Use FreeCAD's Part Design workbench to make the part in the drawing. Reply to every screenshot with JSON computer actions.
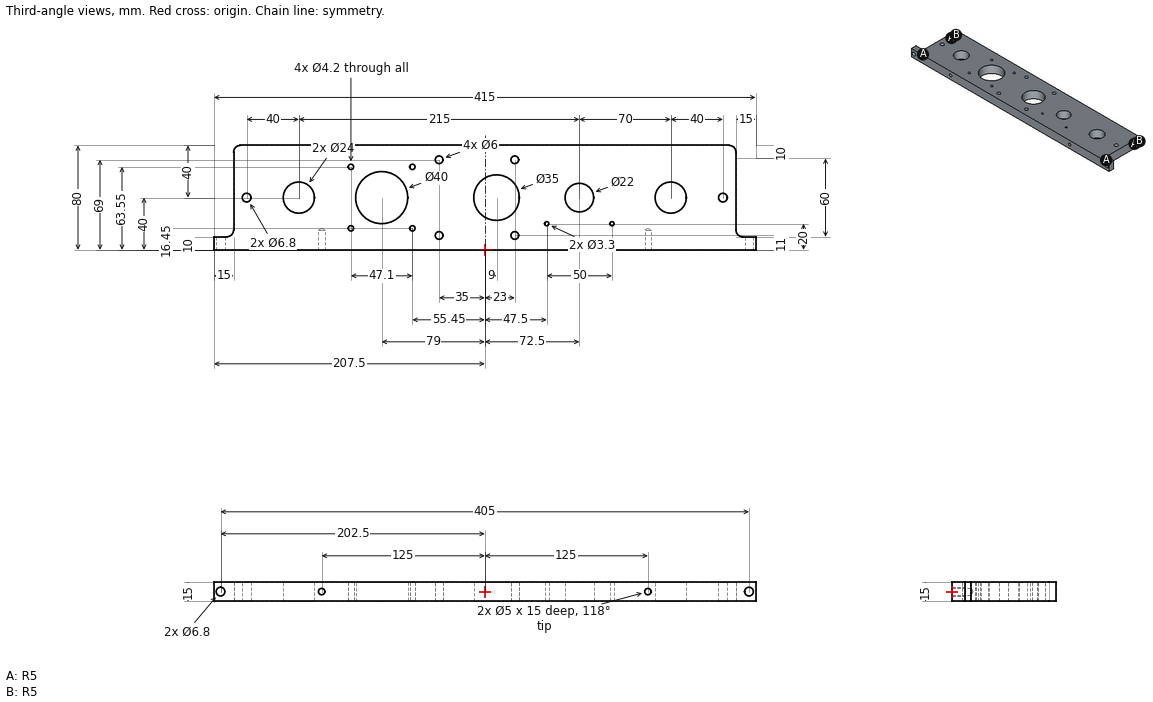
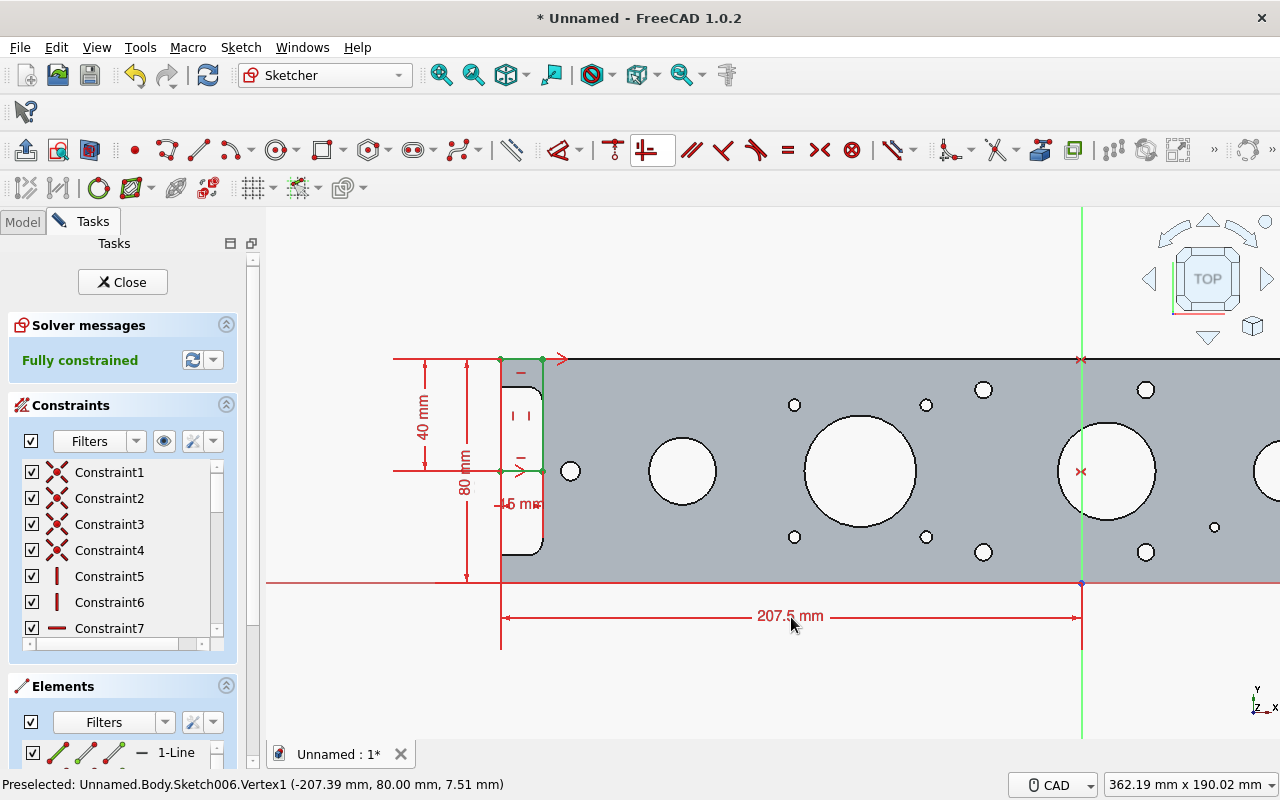
{"action": "left_click", "coordinate": [123, 282]}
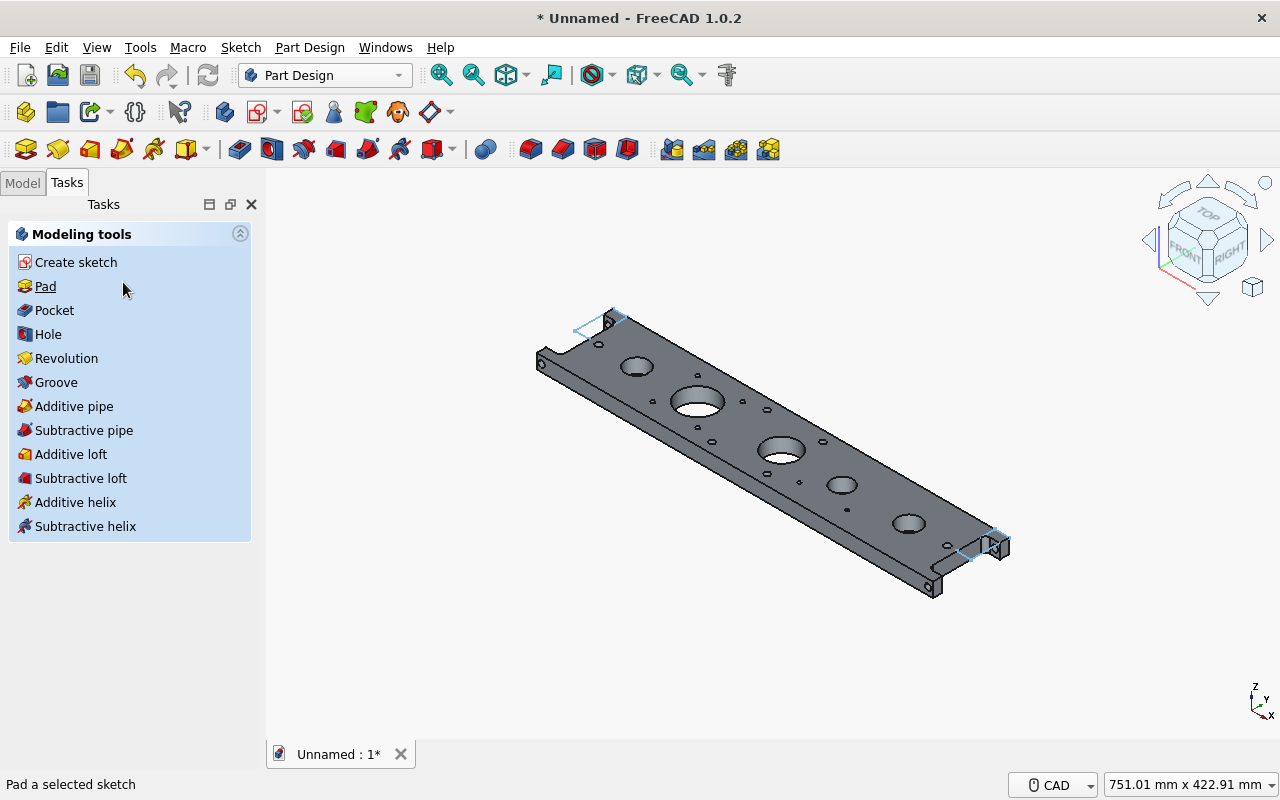
{"action": "left_click", "coordinate": [240, 150]}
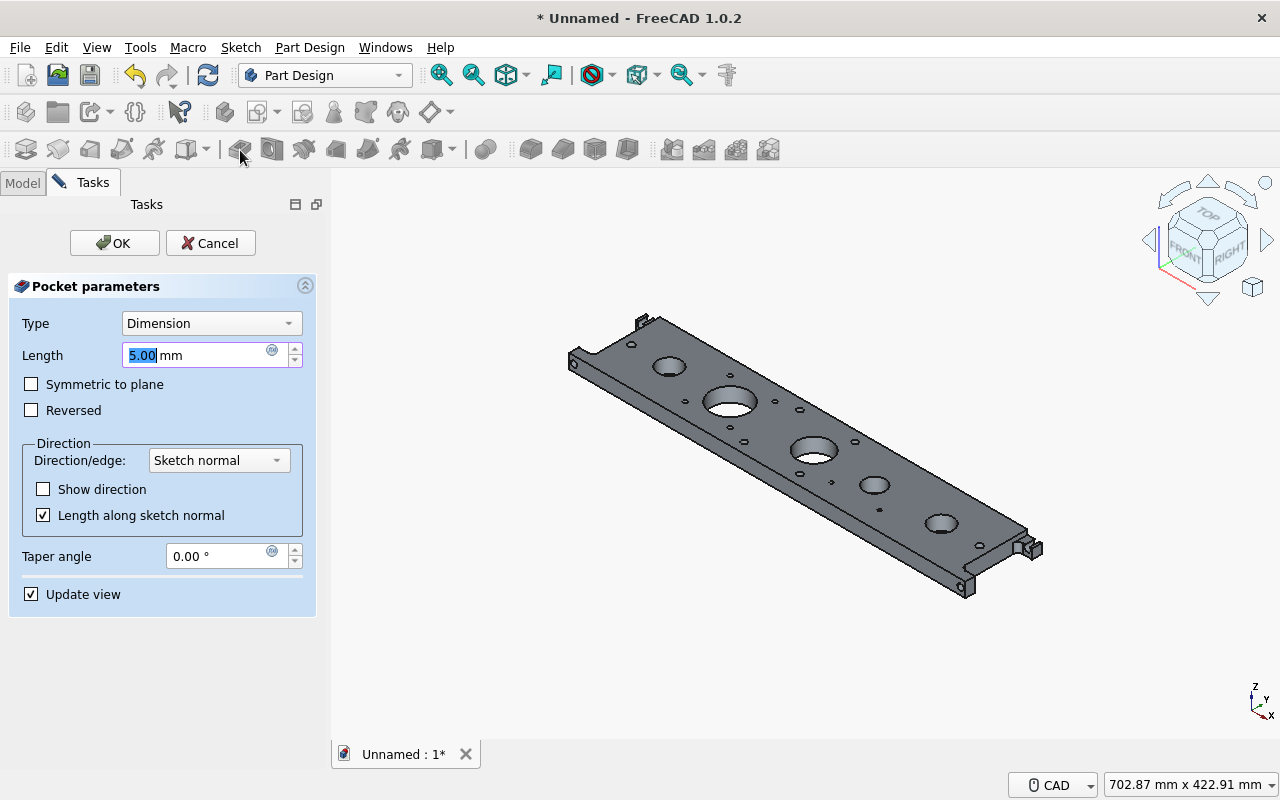
{"action": "left_click", "coordinate": [212, 324]}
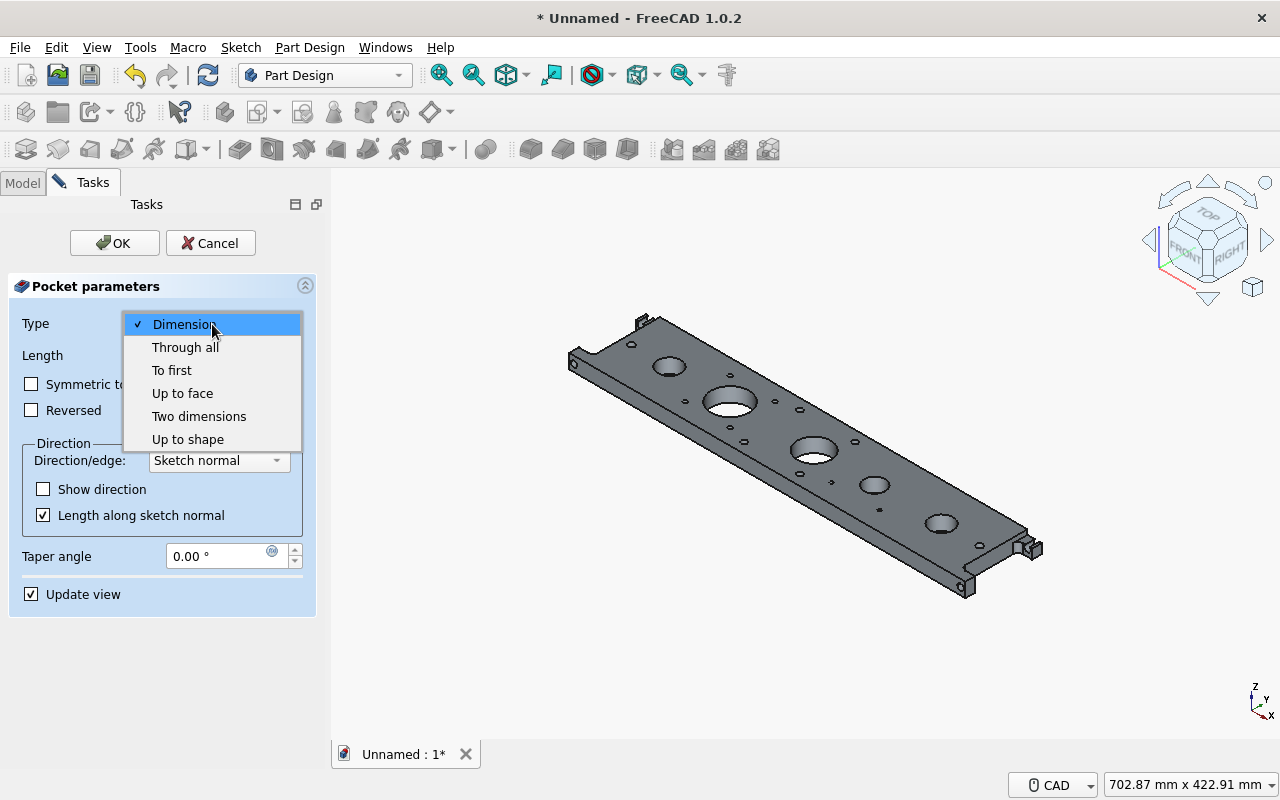
{"action": "left_click", "coordinate": [212, 348]}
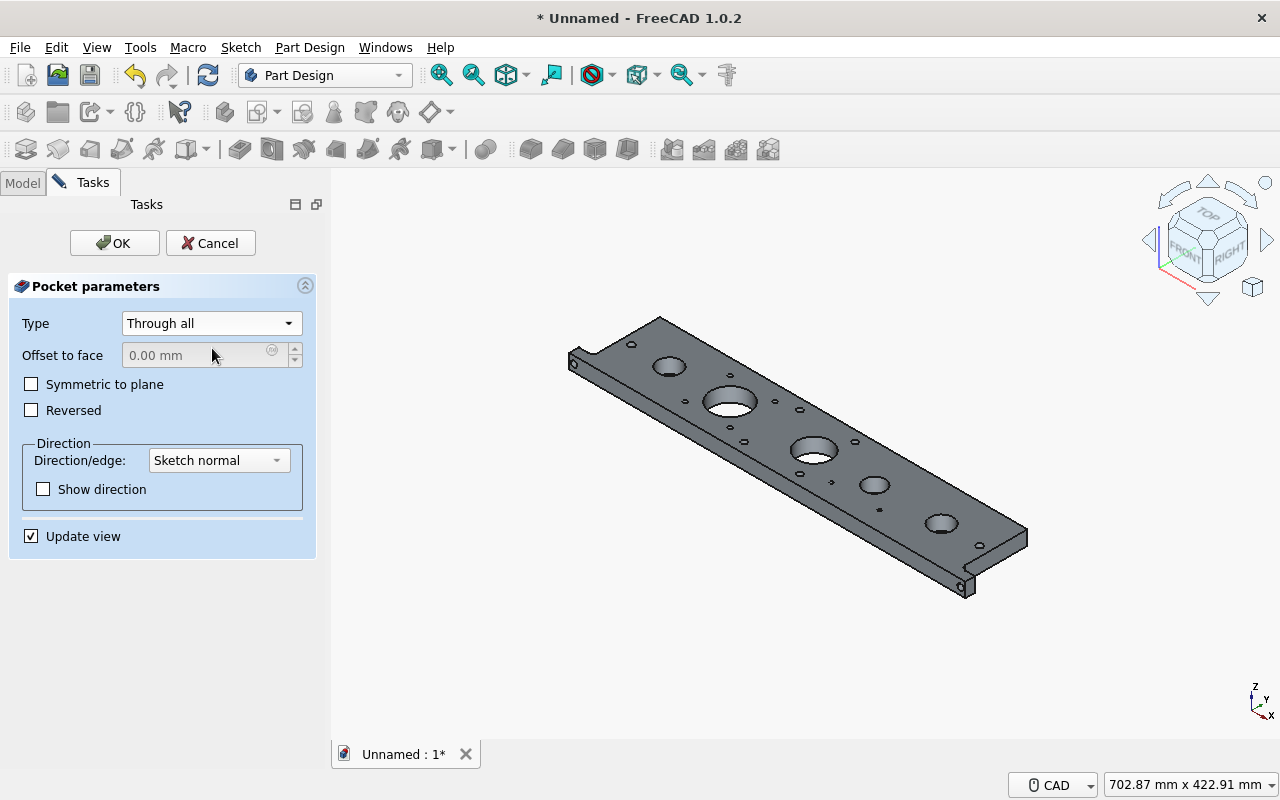
{"action": "left_click", "coordinate": [115, 243]}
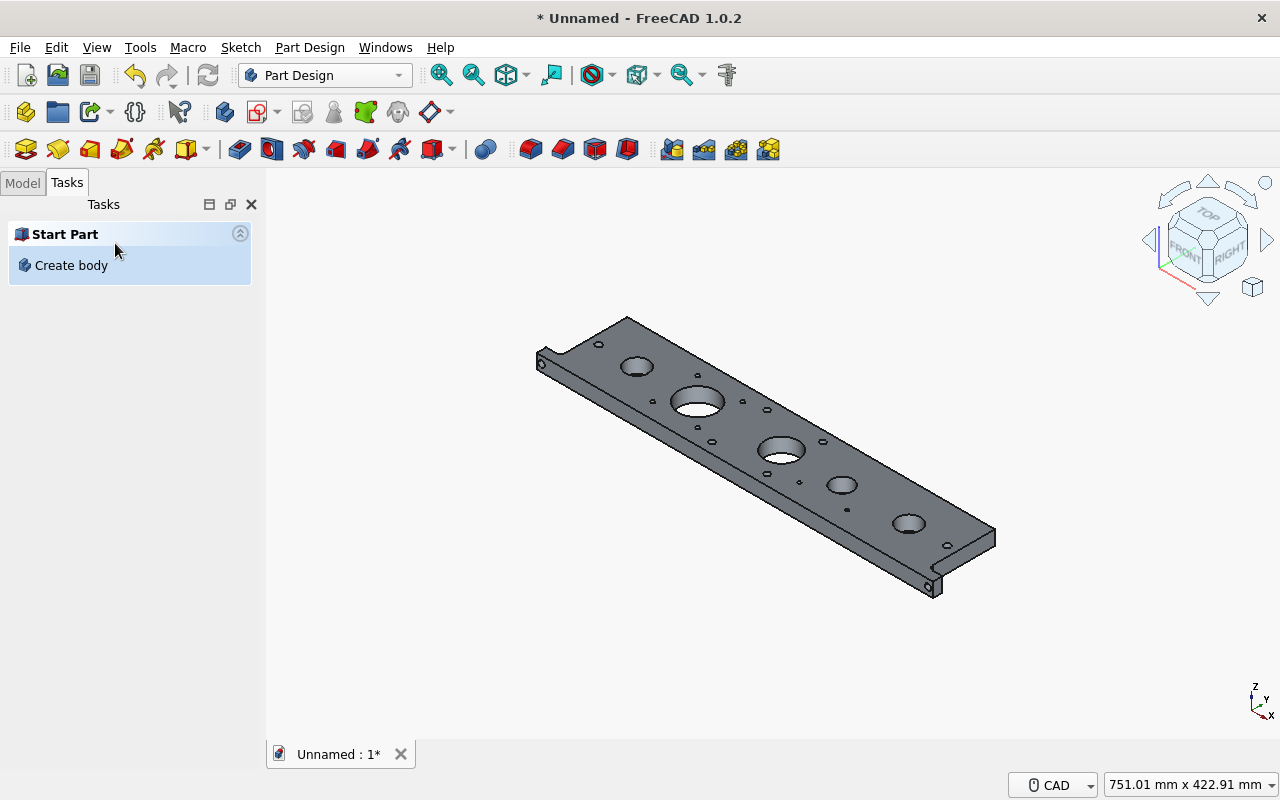
{"action": "scroll", "coordinate": [627, 324], "scroll_direction": "up", "scroll_amount": 4}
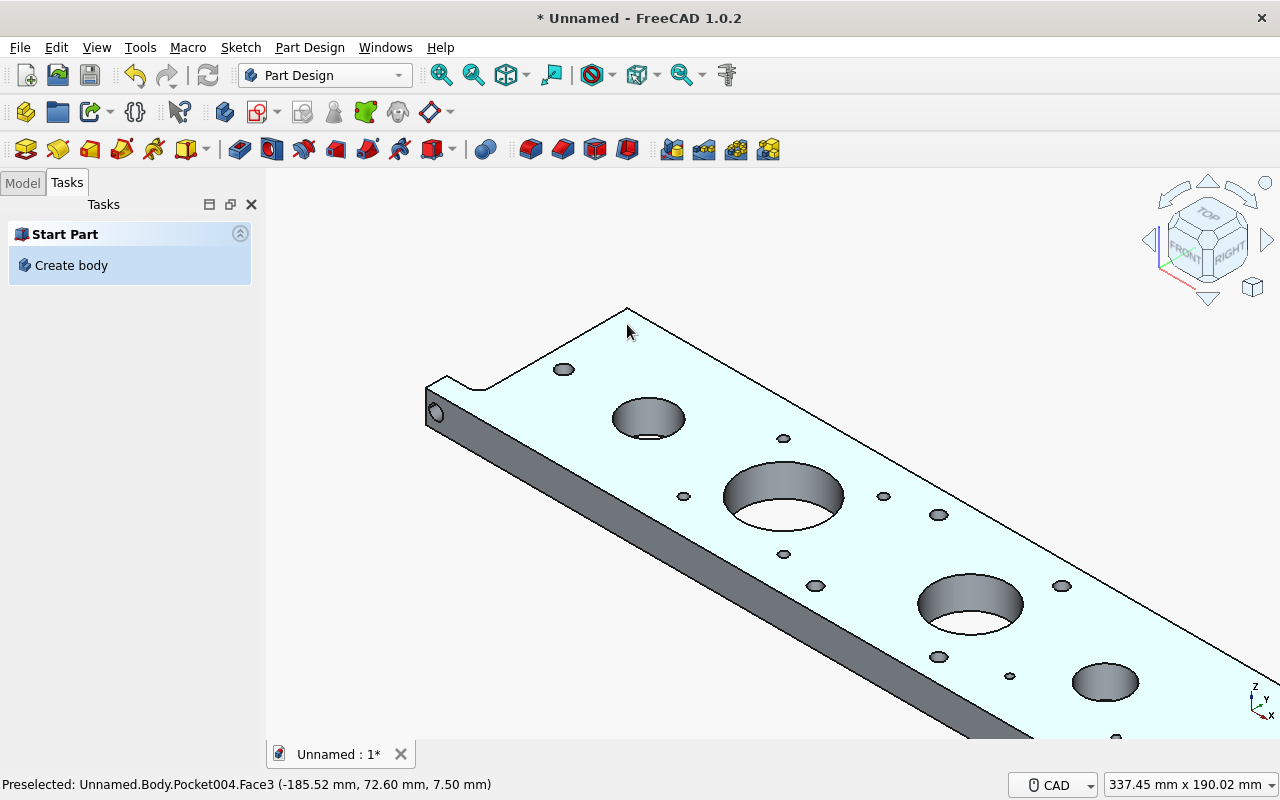
{"action": "left_click", "coordinate": [442, 76]}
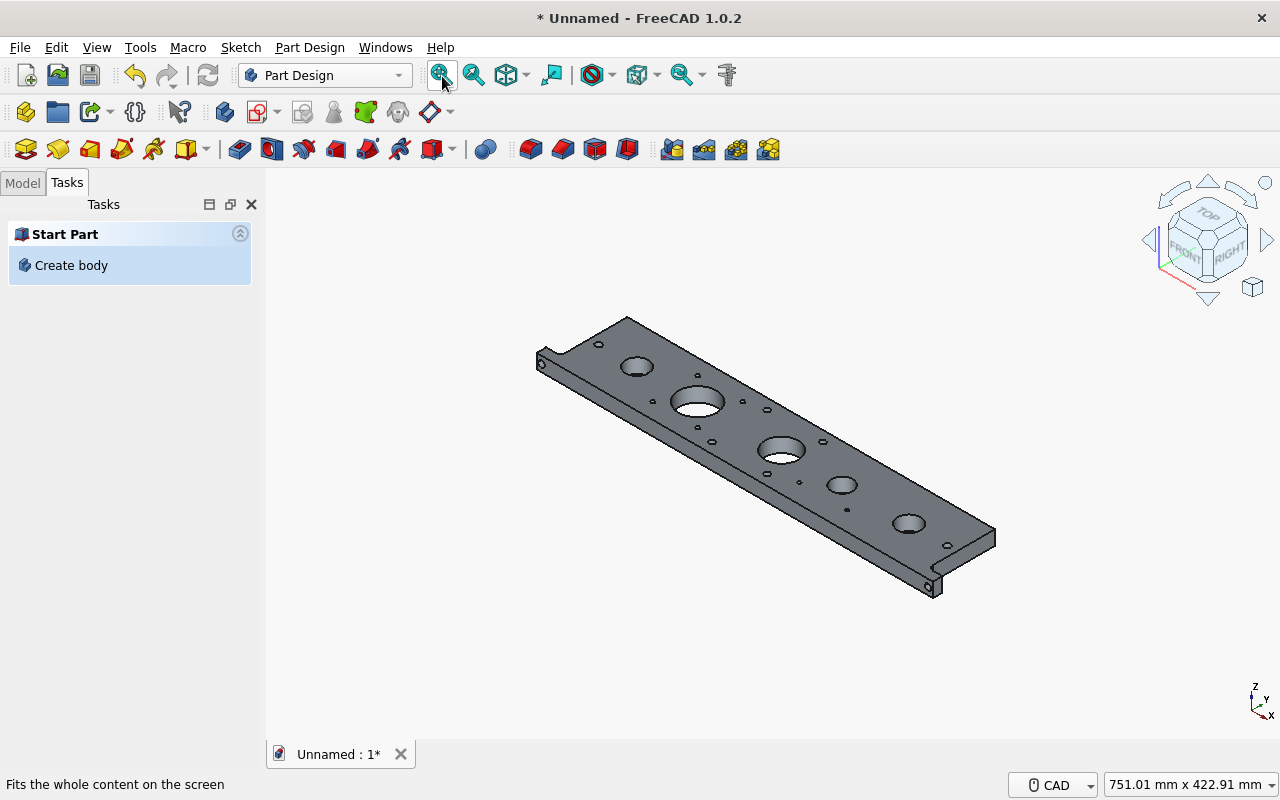
{"action": "key", "text": "2"}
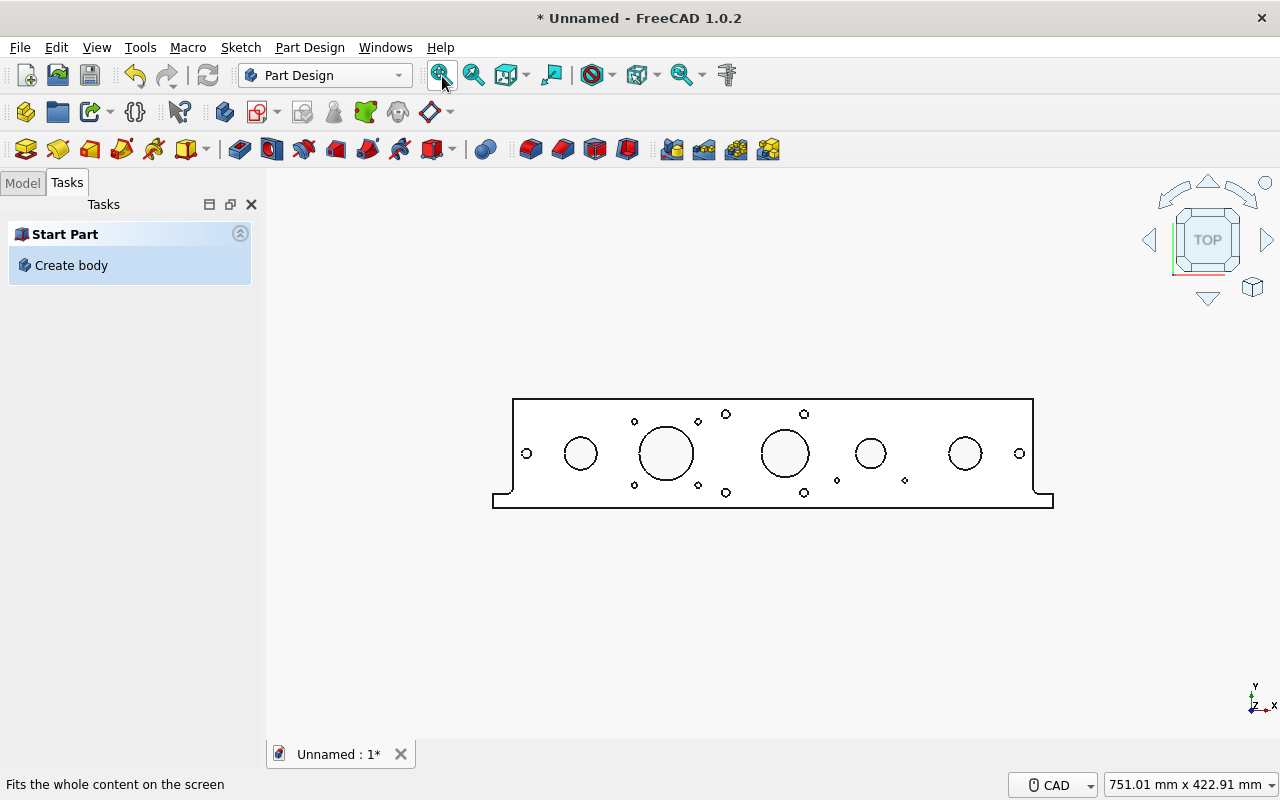
{"action": "scroll", "coordinate": [513, 398], "scroll_direction": "up", "scroll_amount": 4}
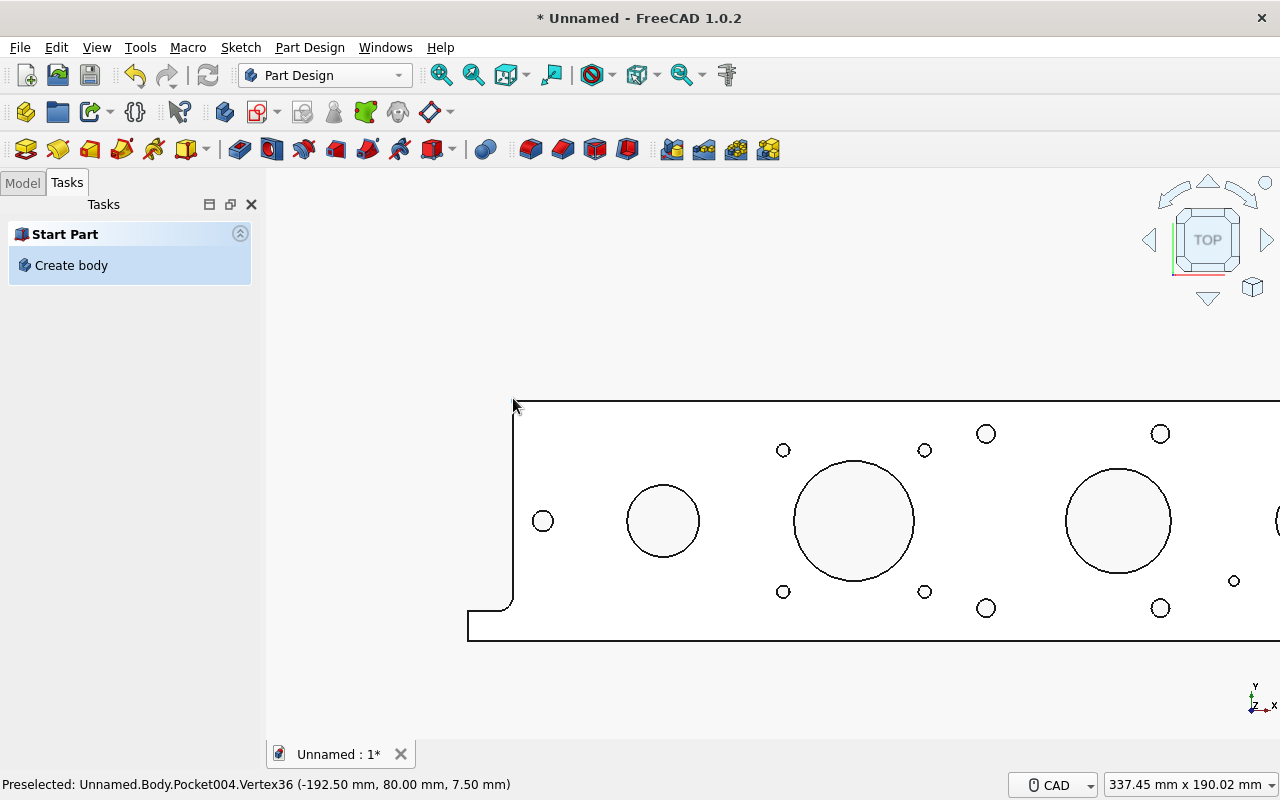
{"action": "left_click", "coordinate": [442, 76]}